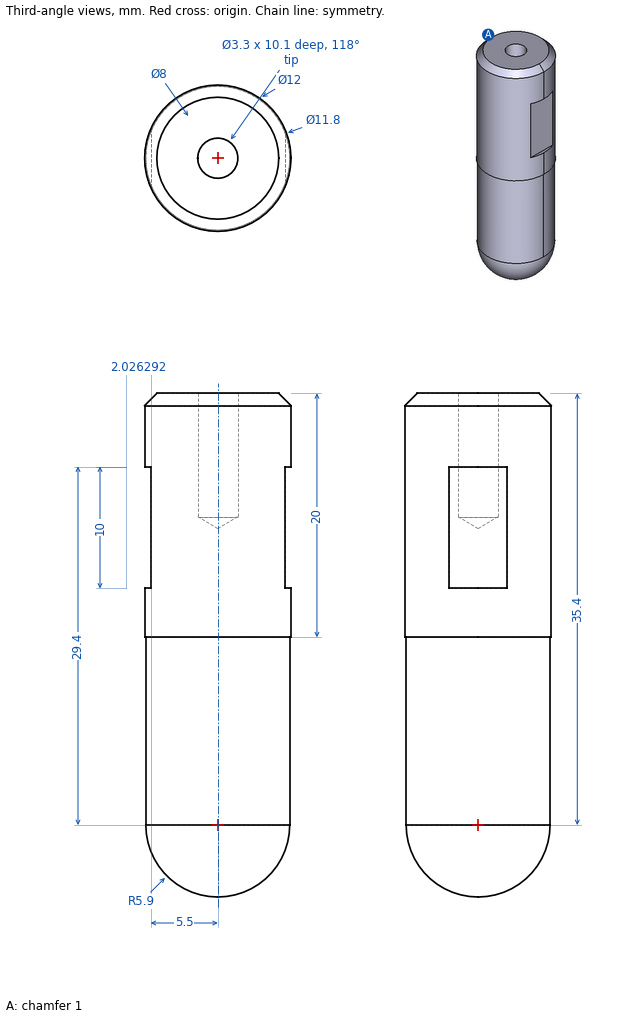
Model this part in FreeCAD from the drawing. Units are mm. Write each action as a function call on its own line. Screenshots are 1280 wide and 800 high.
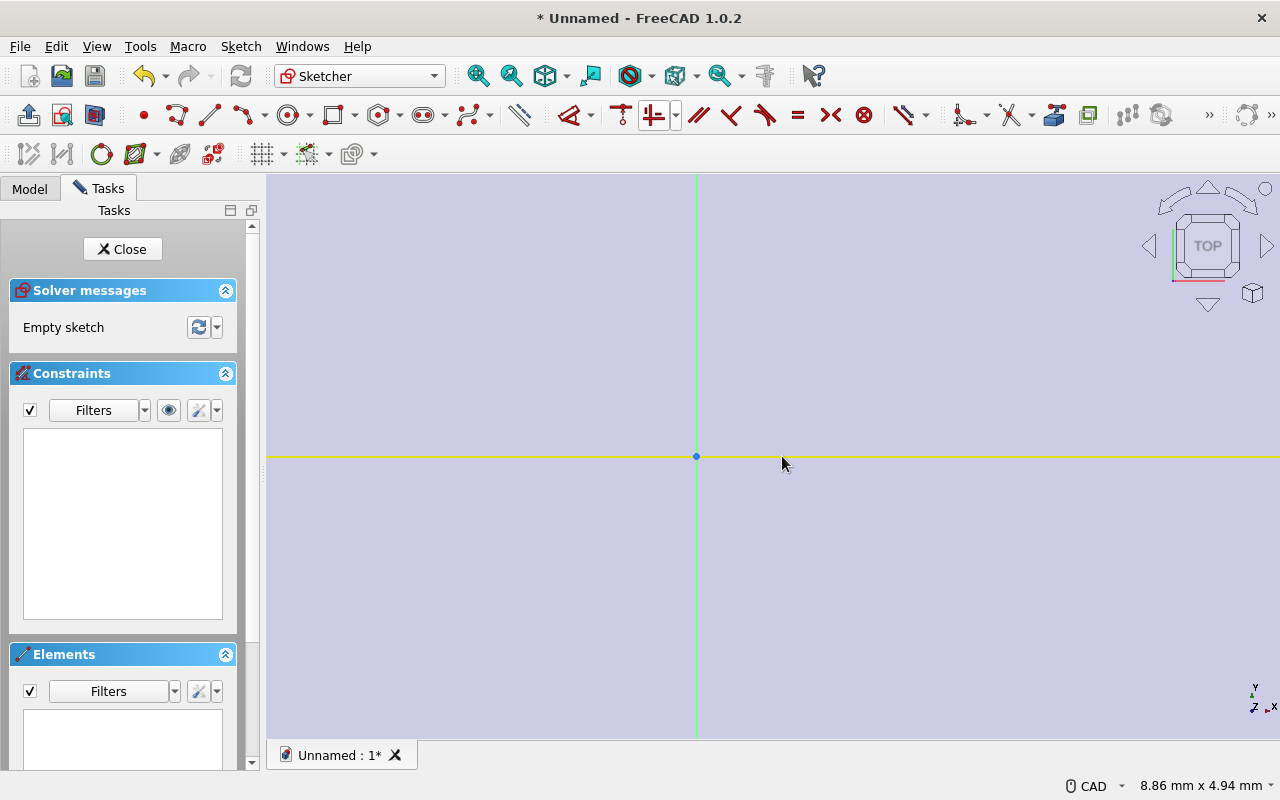
click(288, 116)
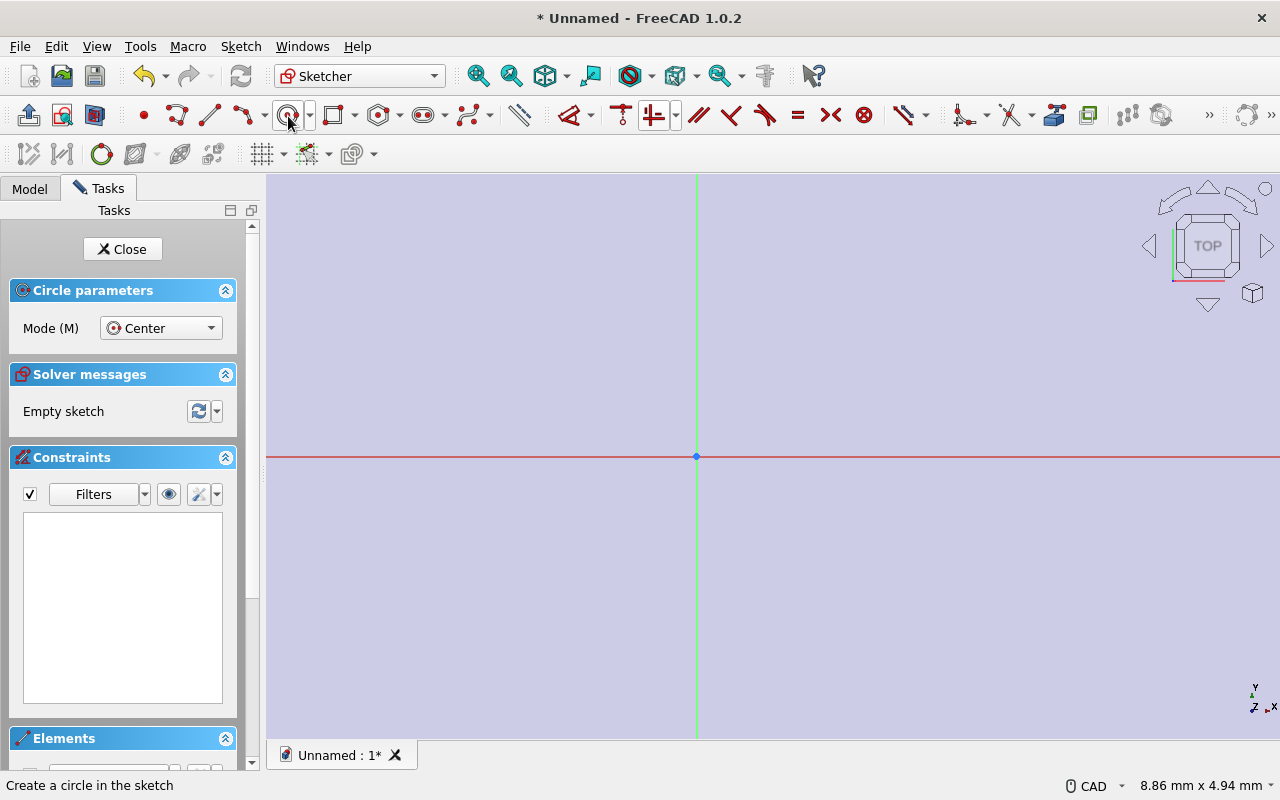
click(697, 456)
click(830, 323)
key(Escape)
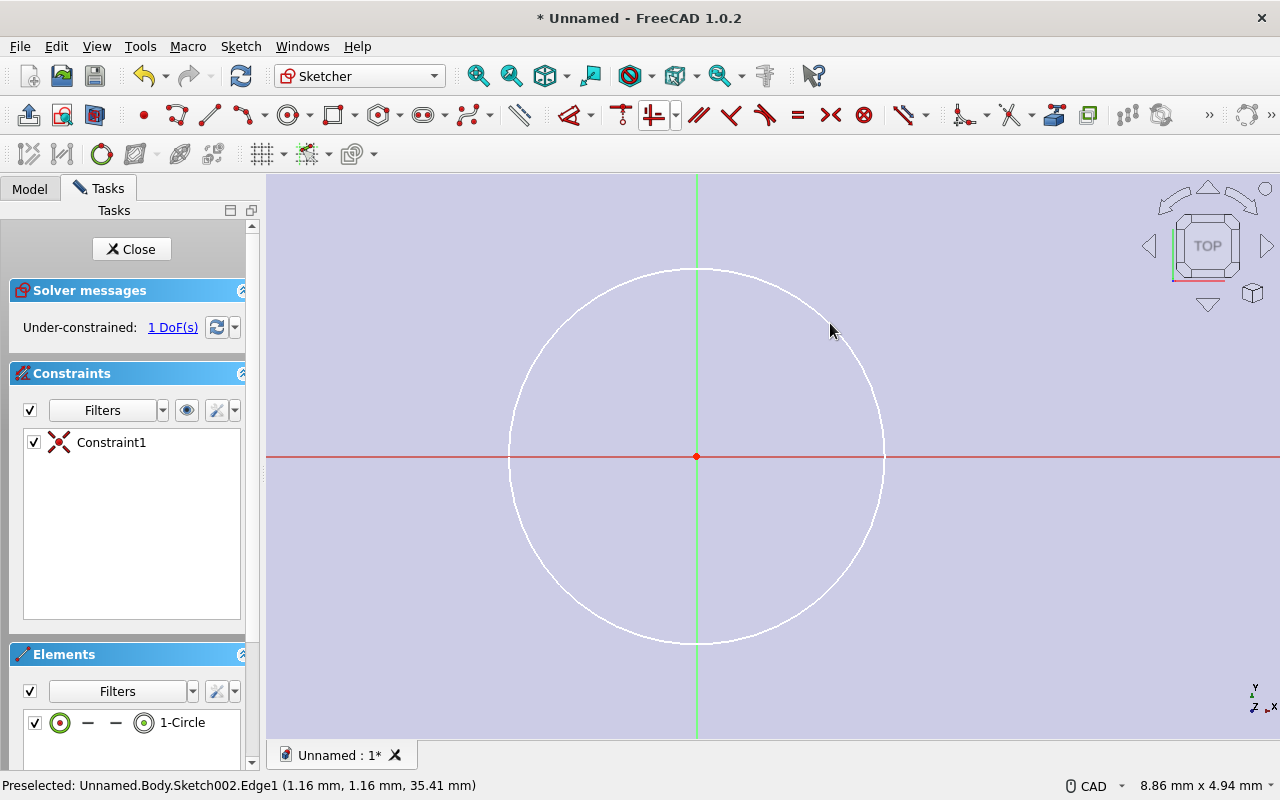
click(568, 116)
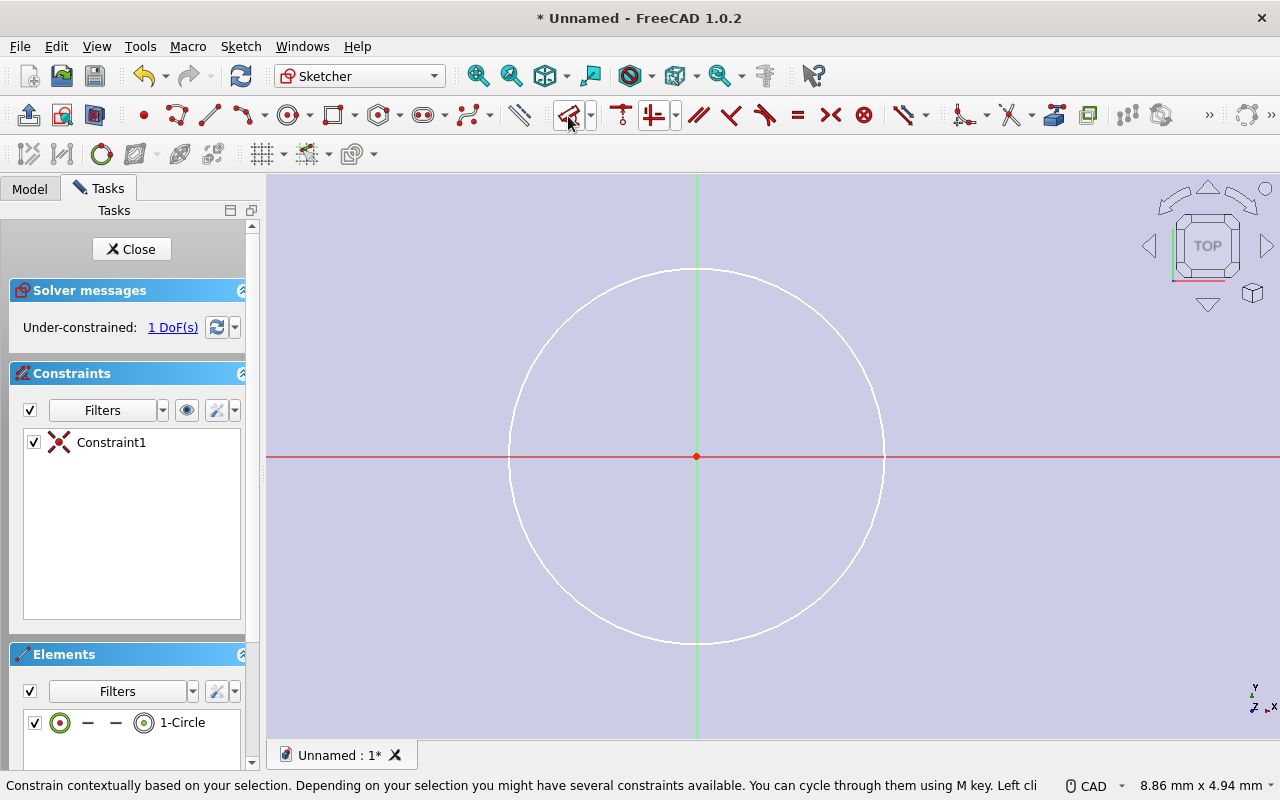
click(829, 323)
click(852, 300)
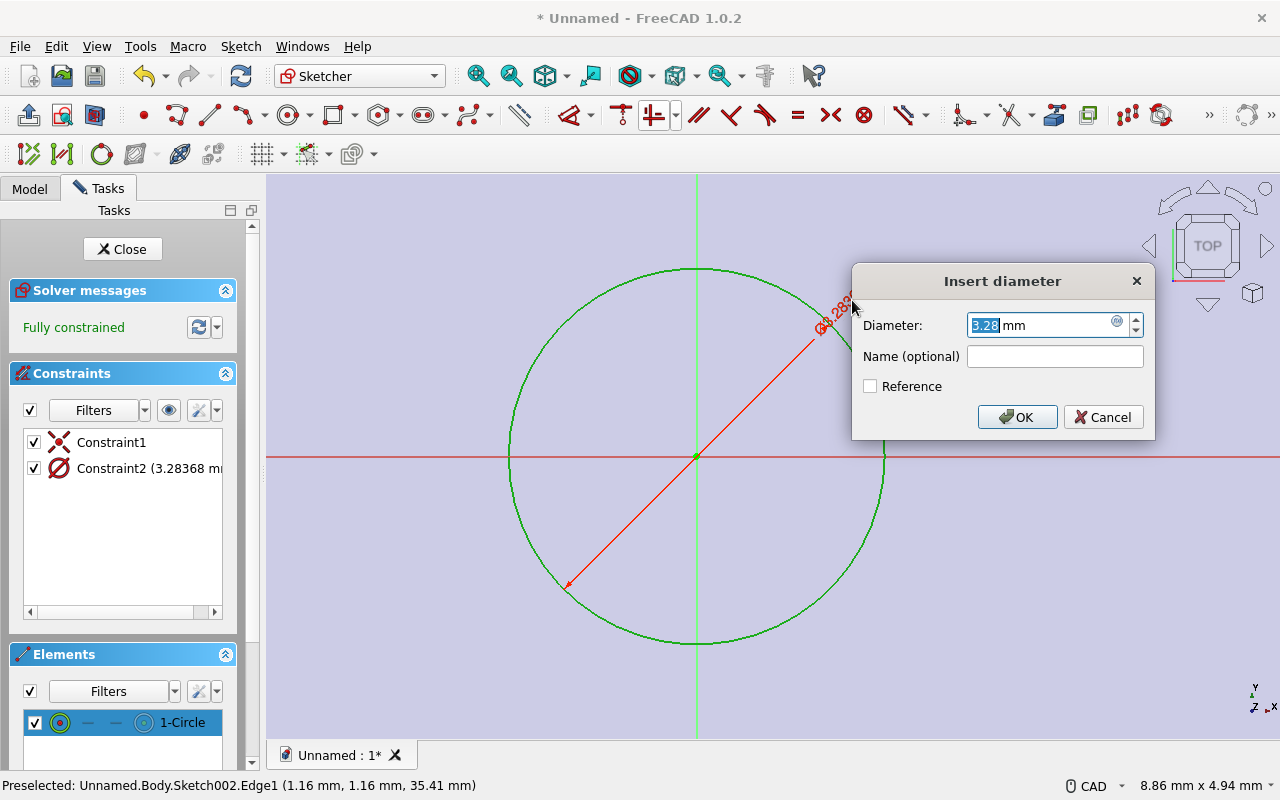
text(3.3)
key(Return)
key(Escape)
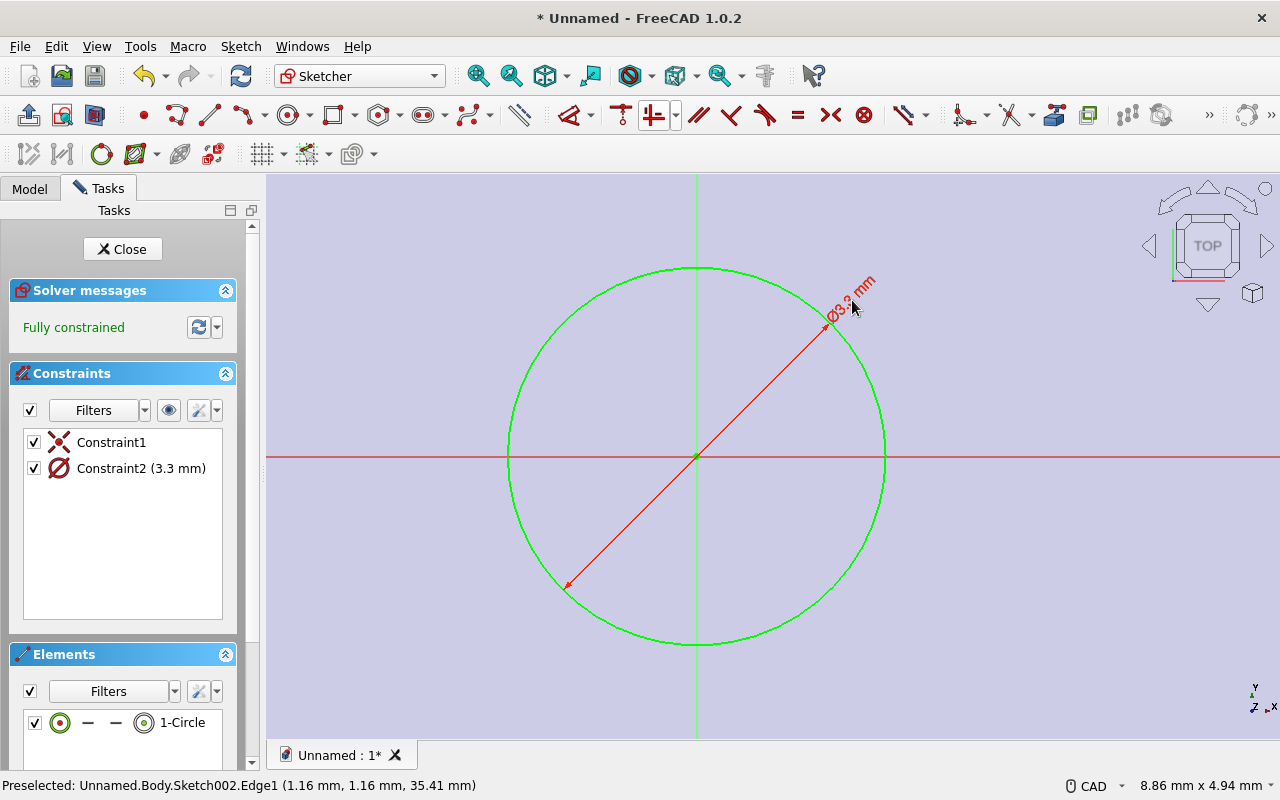
click(123, 249)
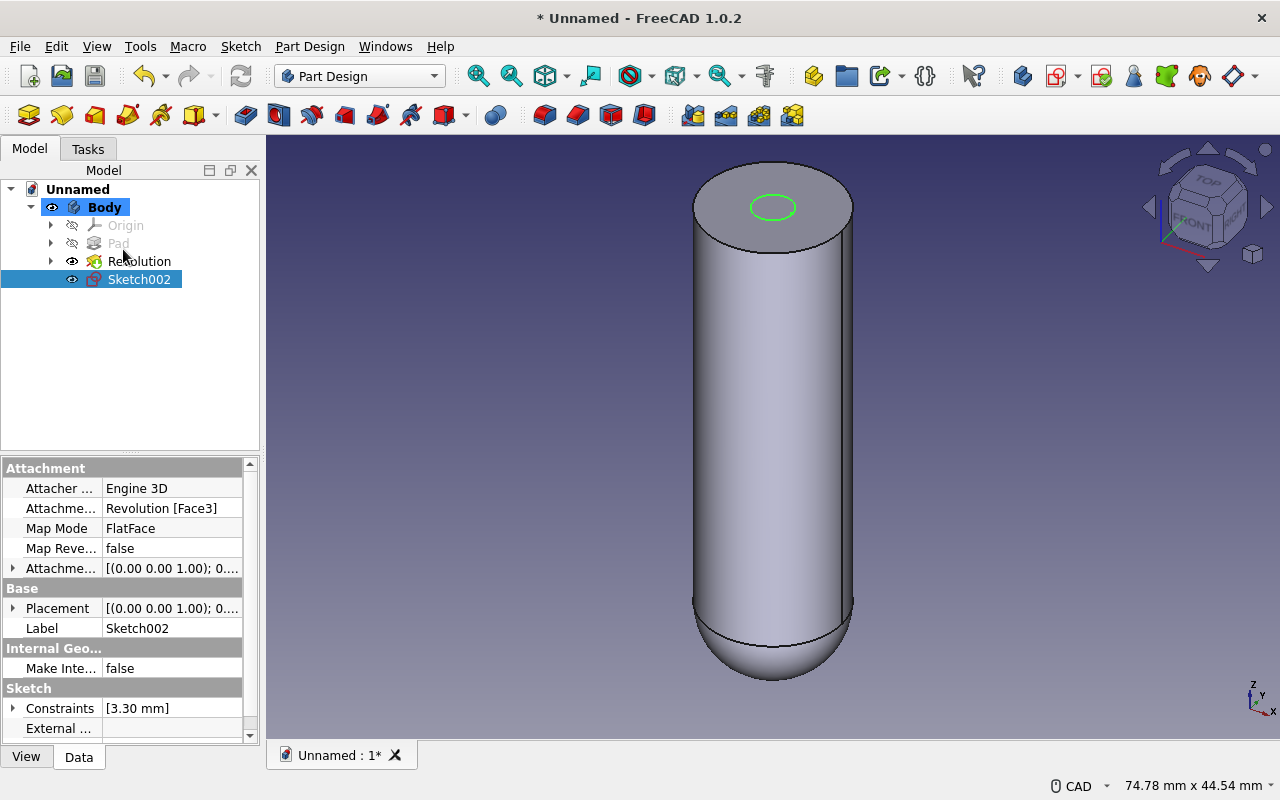
click(279, 116)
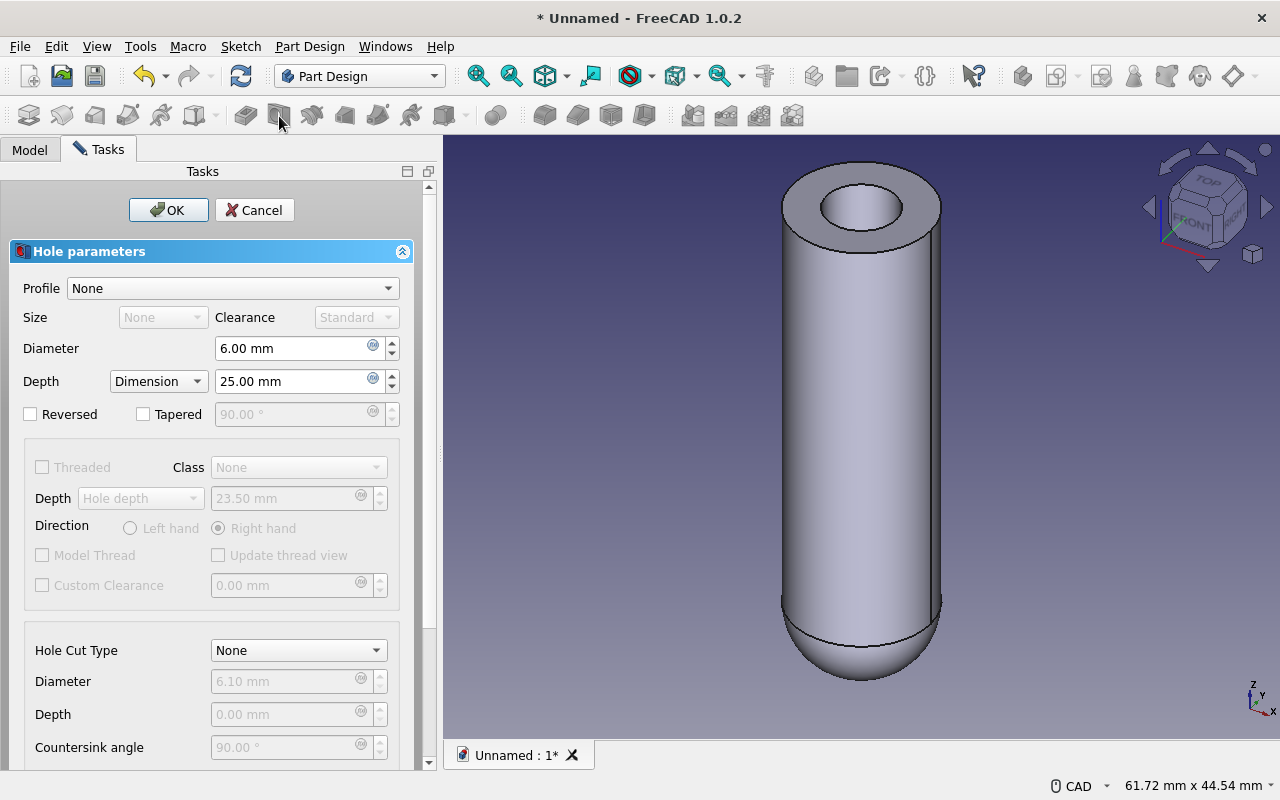
triple_click(300, 348)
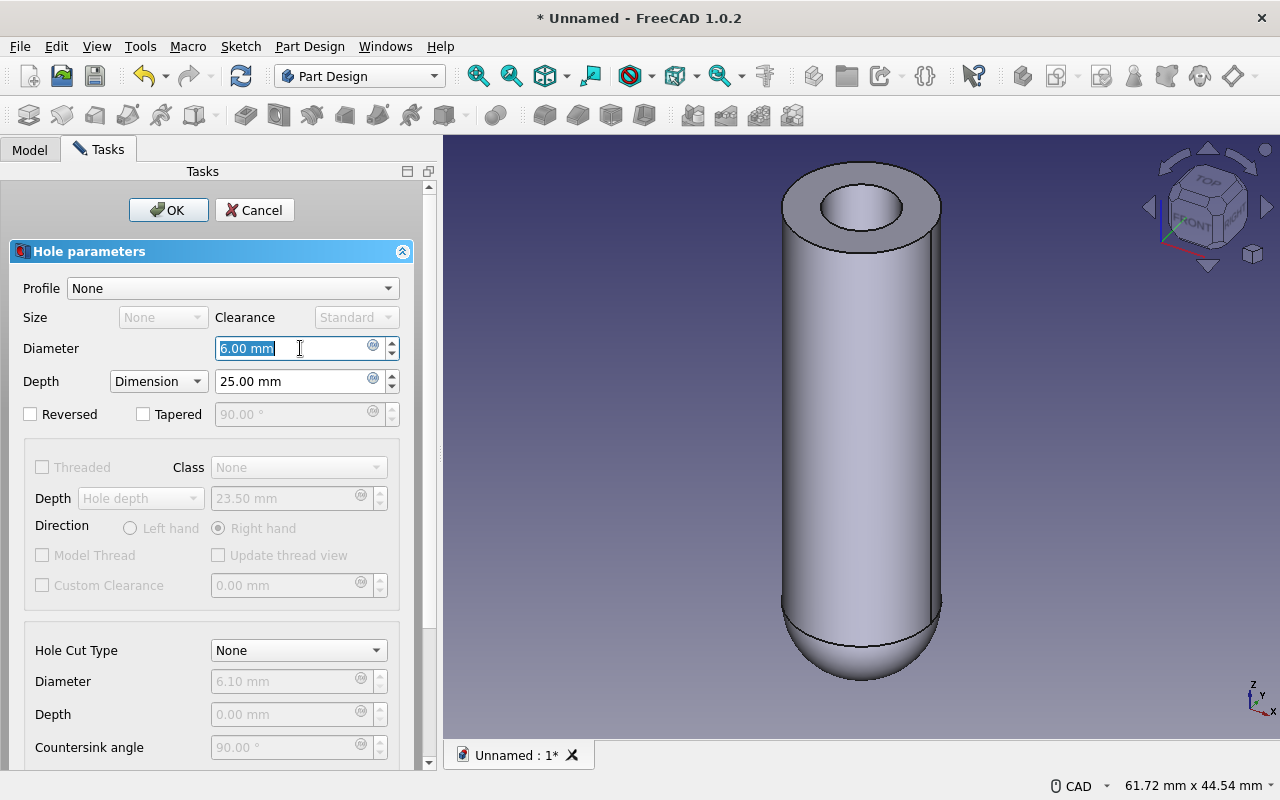
text(3.3)
key(Tab)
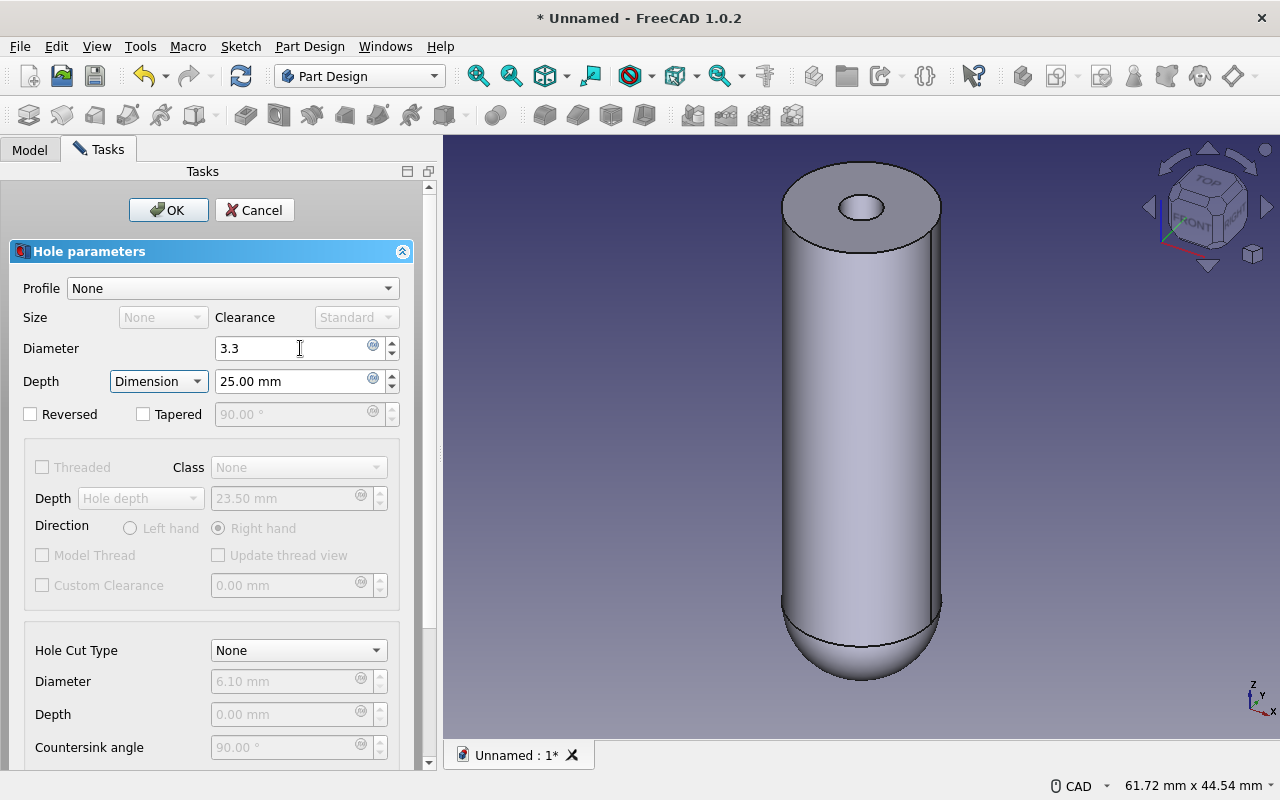
triple_click(300, 382)